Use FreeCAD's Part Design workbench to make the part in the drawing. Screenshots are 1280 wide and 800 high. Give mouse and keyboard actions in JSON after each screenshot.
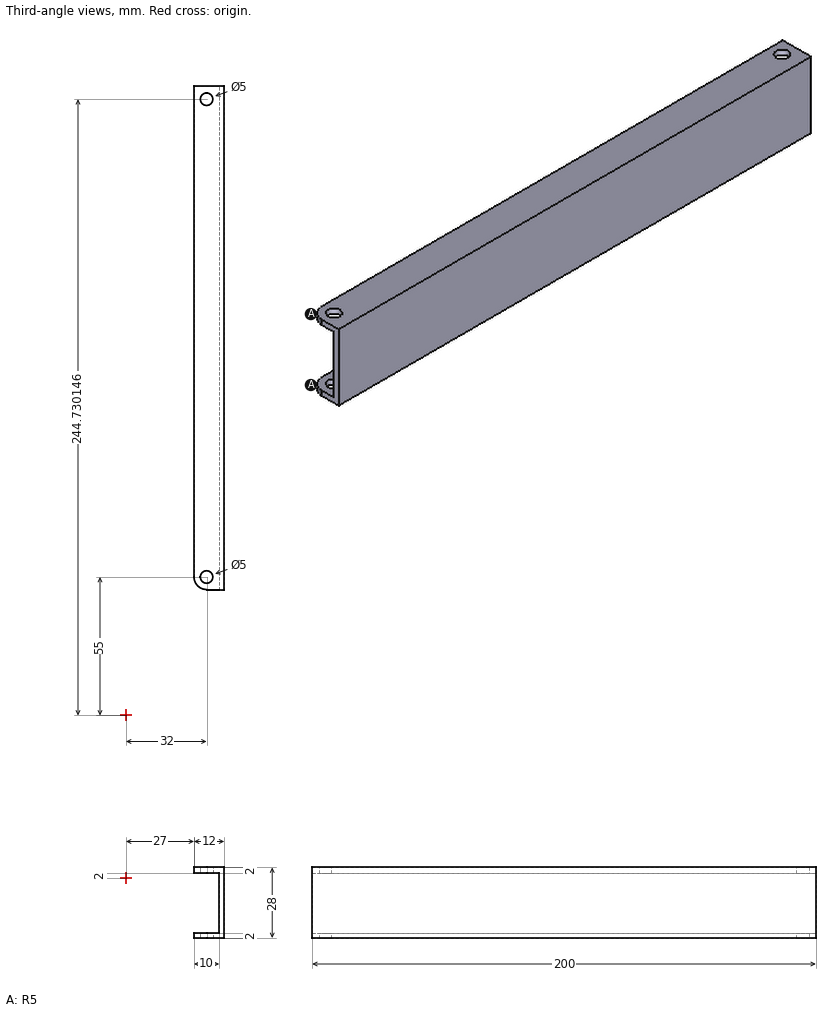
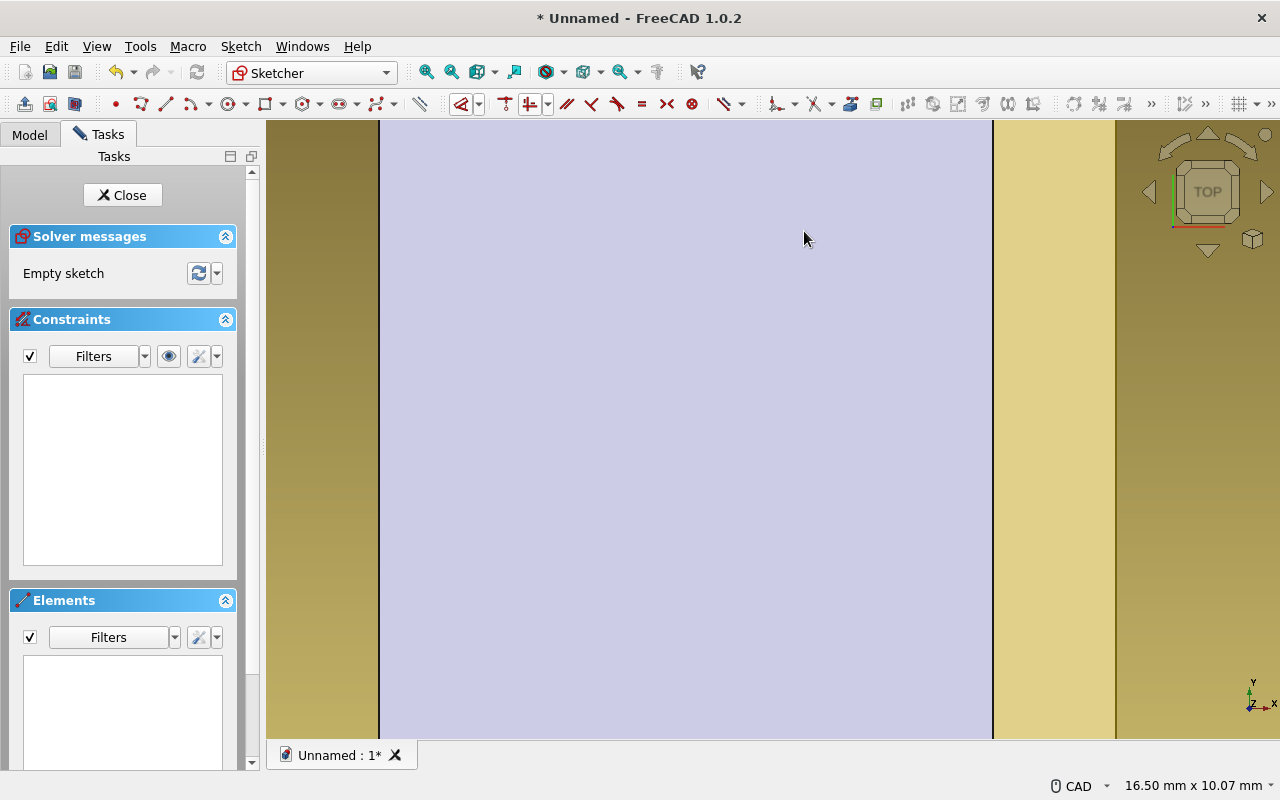
{"action": "left_click", "coordinate": [228, 104]}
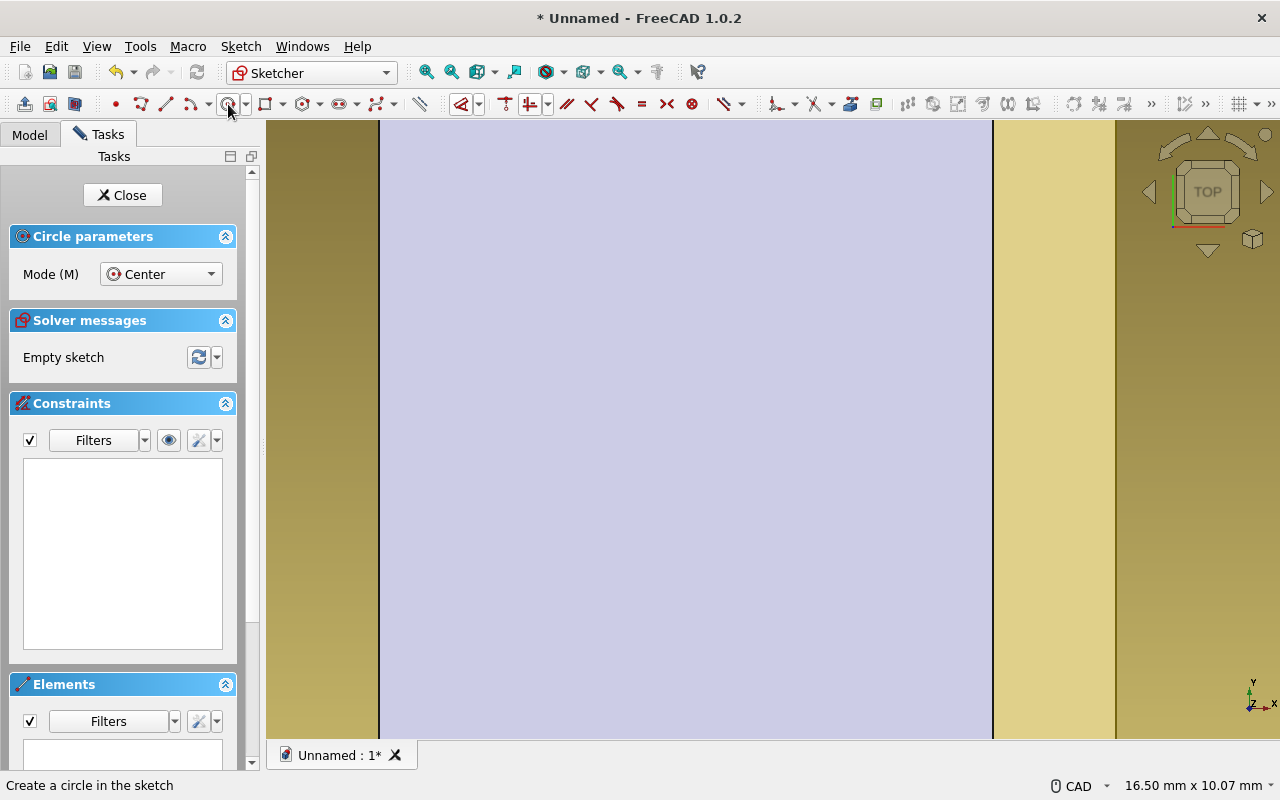
{"action": "left_click", "coordinate": [686, 425]}
{"action": "left_click", "coordinate": [794, 316]}
{"action": "key", "text": "Escape"}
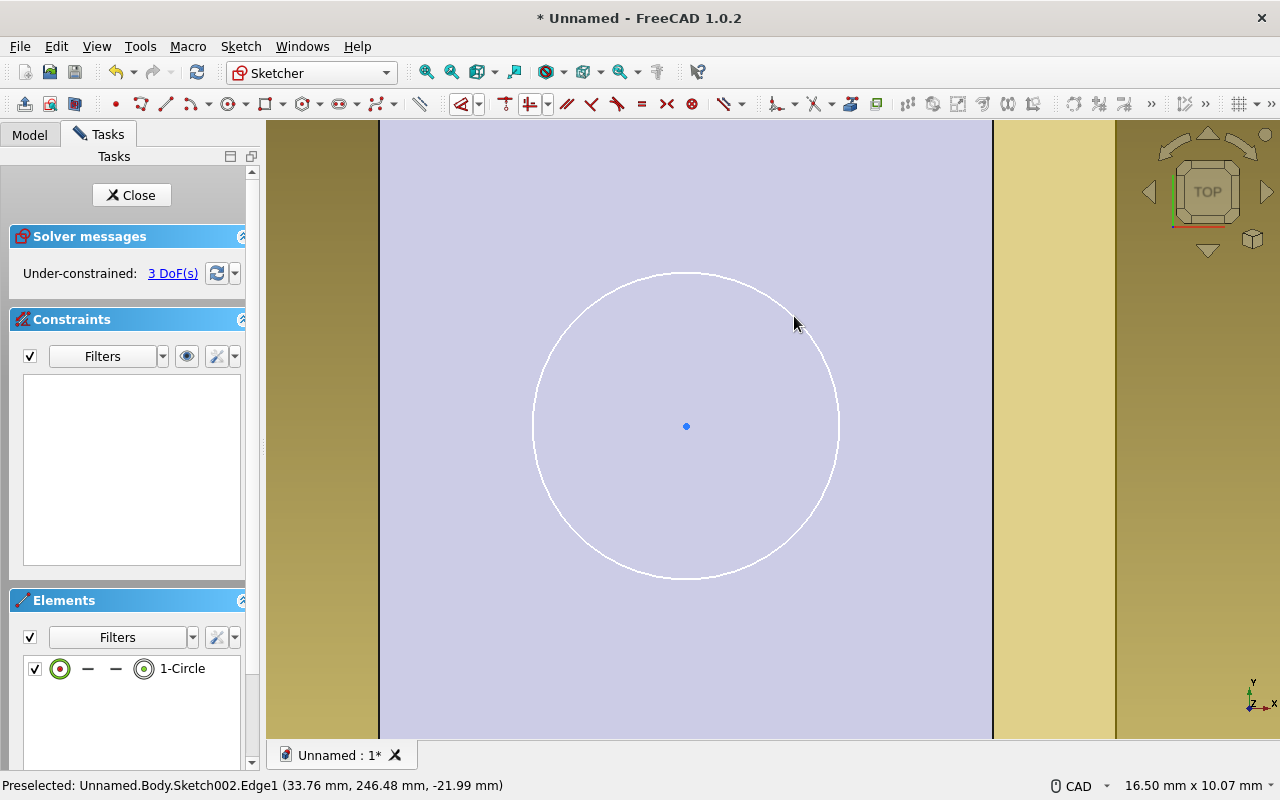
{"action": "left_click", "coordinate": [794, 317]}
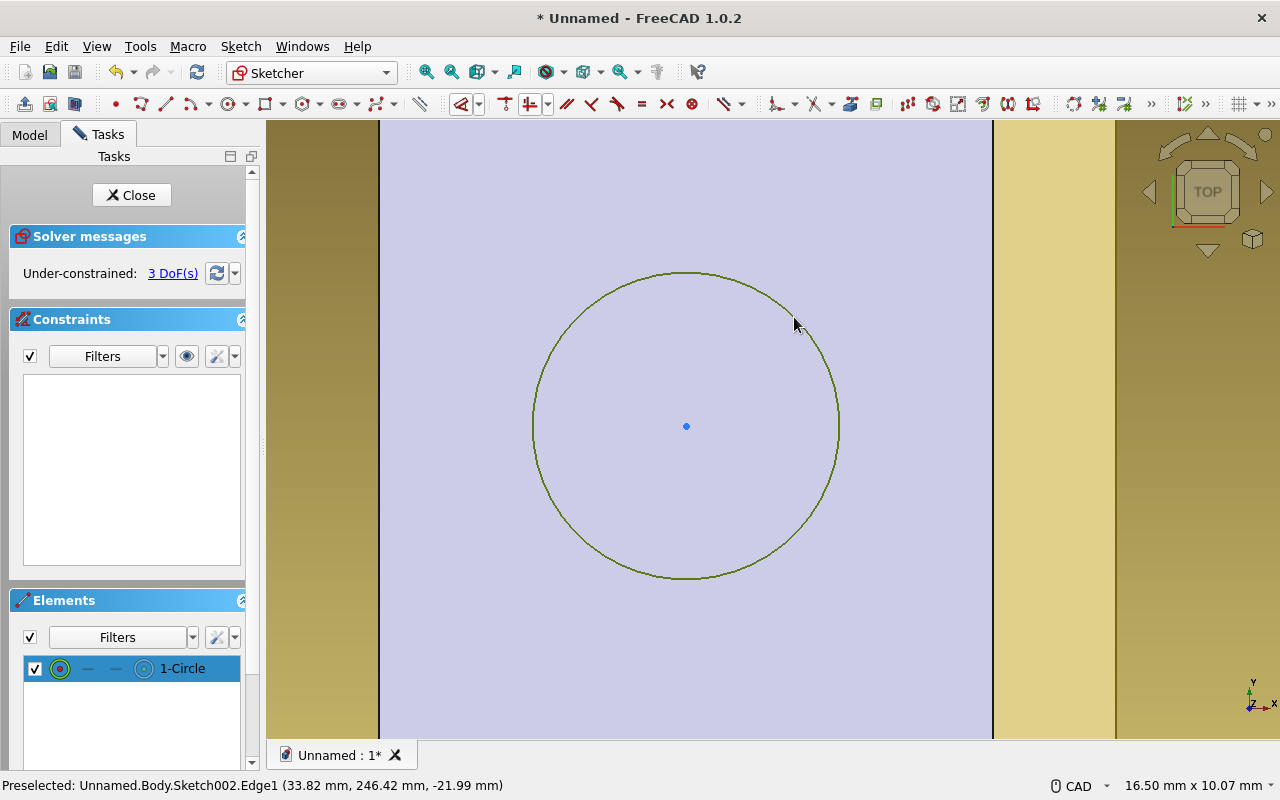
{"action": "key", "text": "k o"}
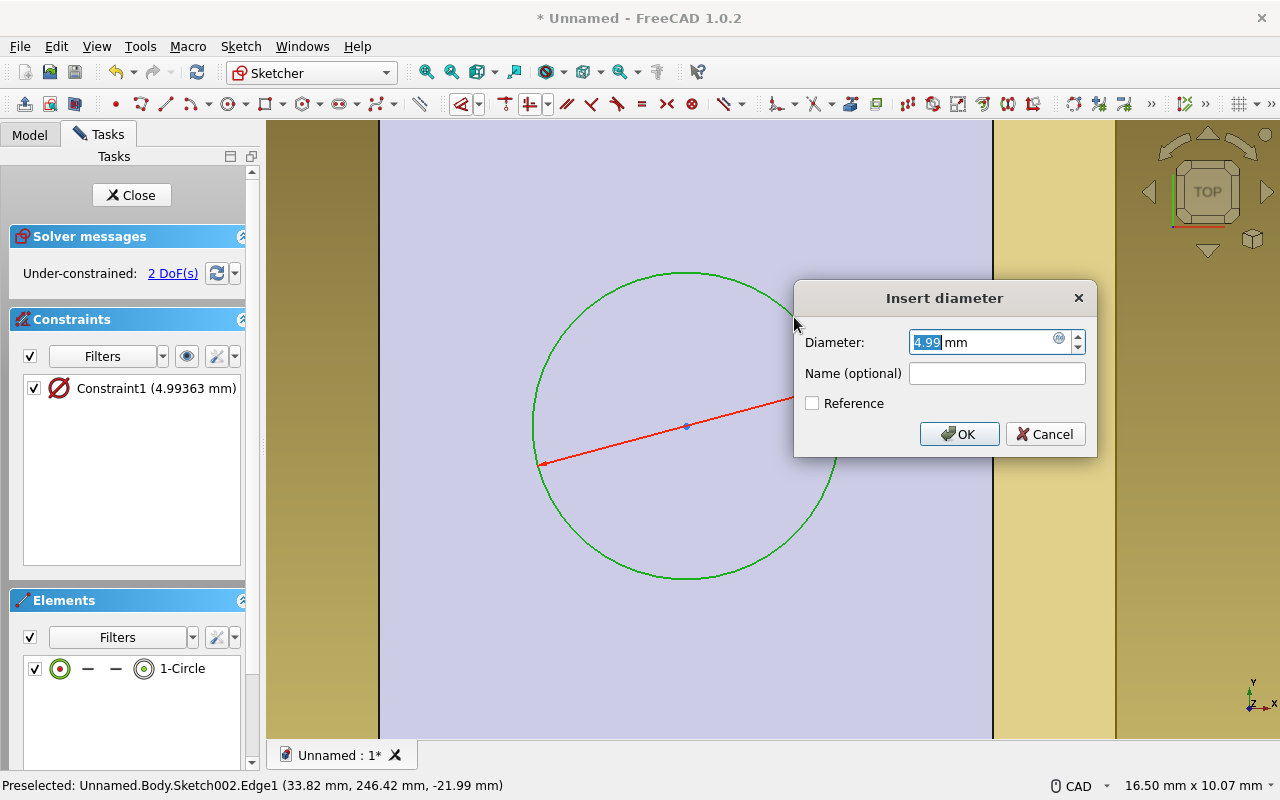
{"action": "type", "text": "5"}
{"action": "key", "text": "Return"}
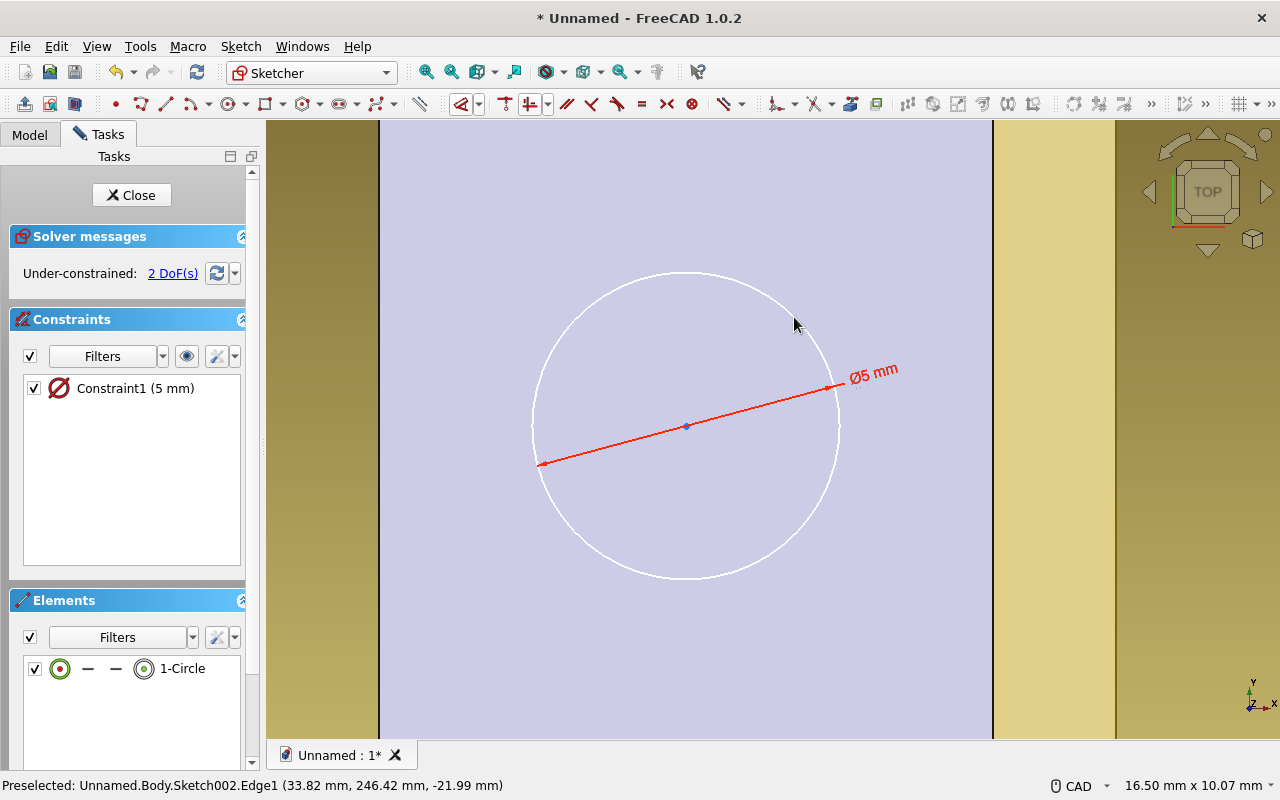
{"action": "left_click", "coordinate": [686, 426]}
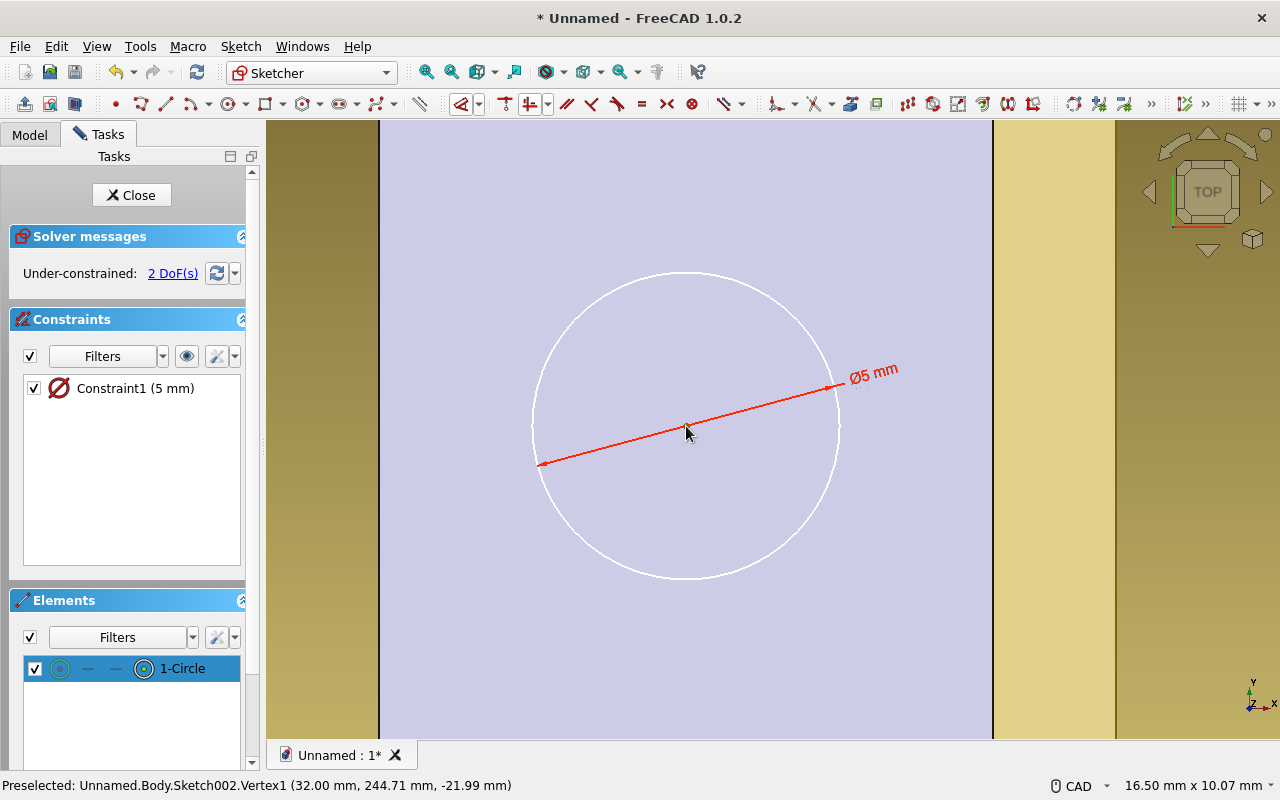
{"action": "key", "text": "l"}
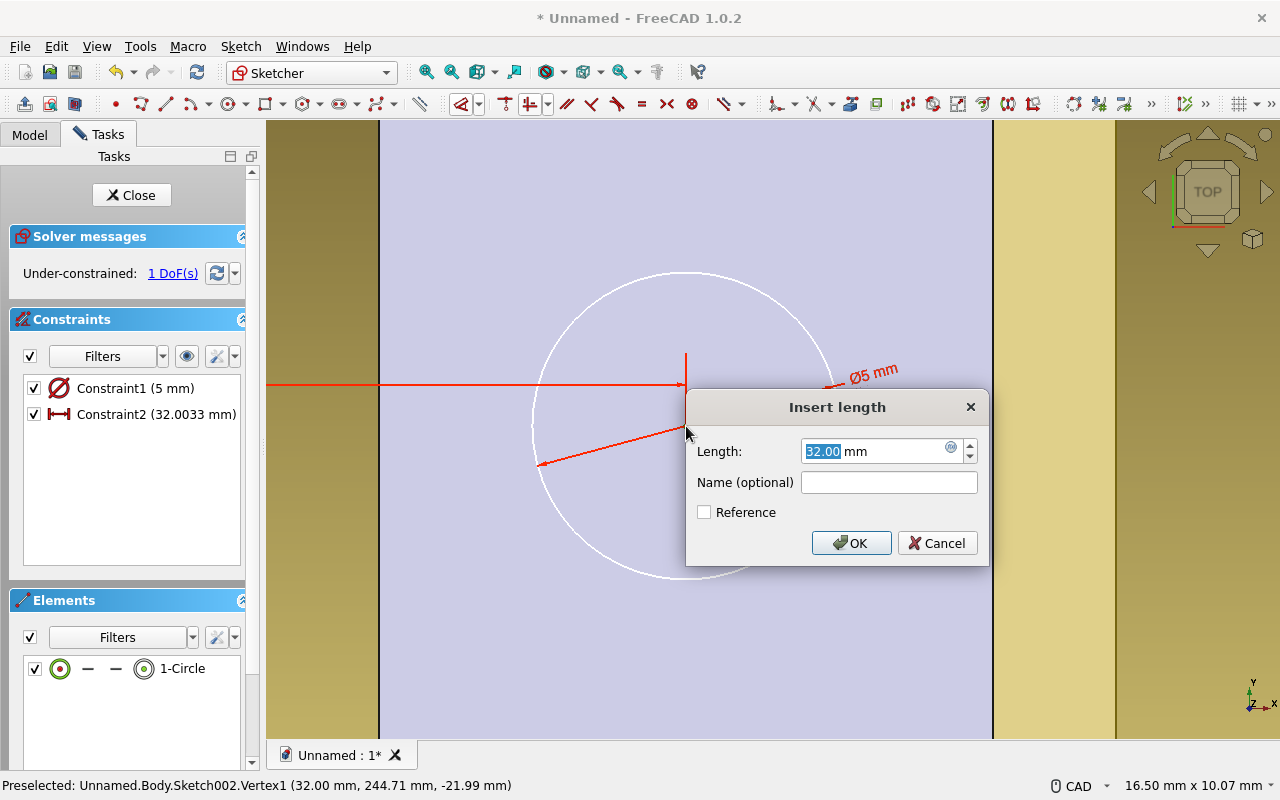
{"action": "type", "text": "32"}
{"action": "key", "text": "Return"}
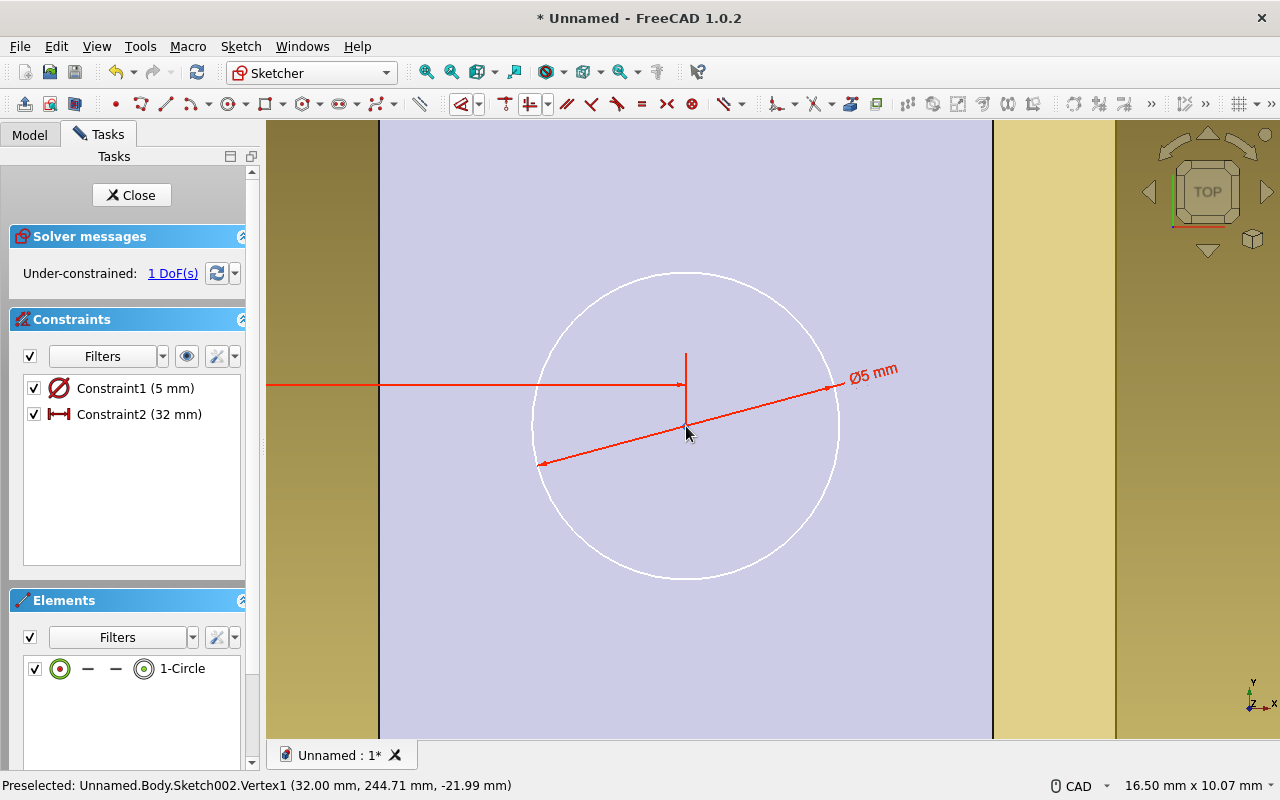
{"action": "left_click", "coordinate": [686, 426]}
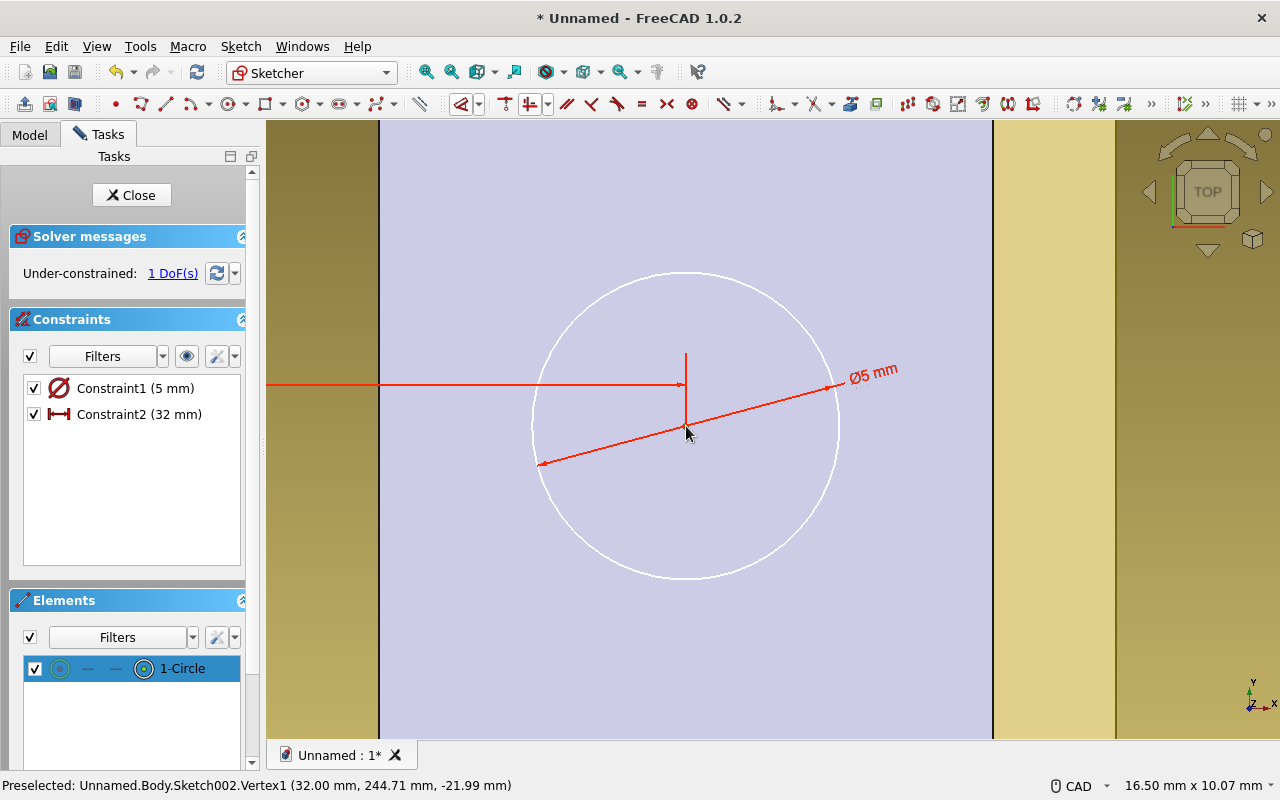
{"action": "left_click", "coordinate": [478, 104]}